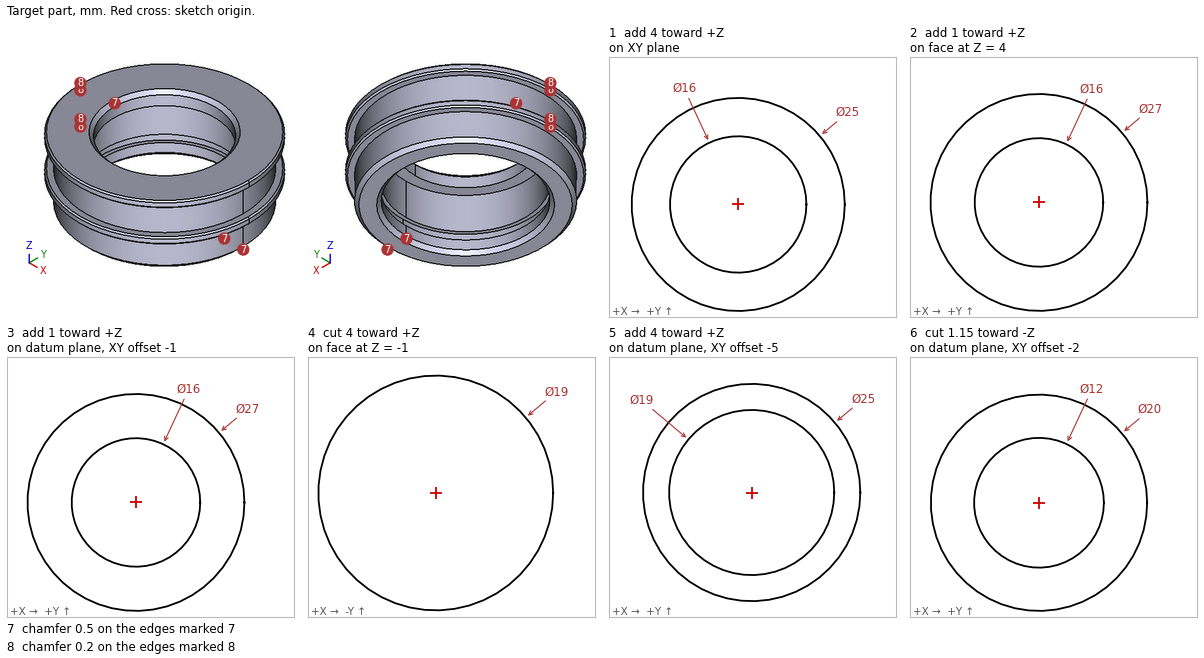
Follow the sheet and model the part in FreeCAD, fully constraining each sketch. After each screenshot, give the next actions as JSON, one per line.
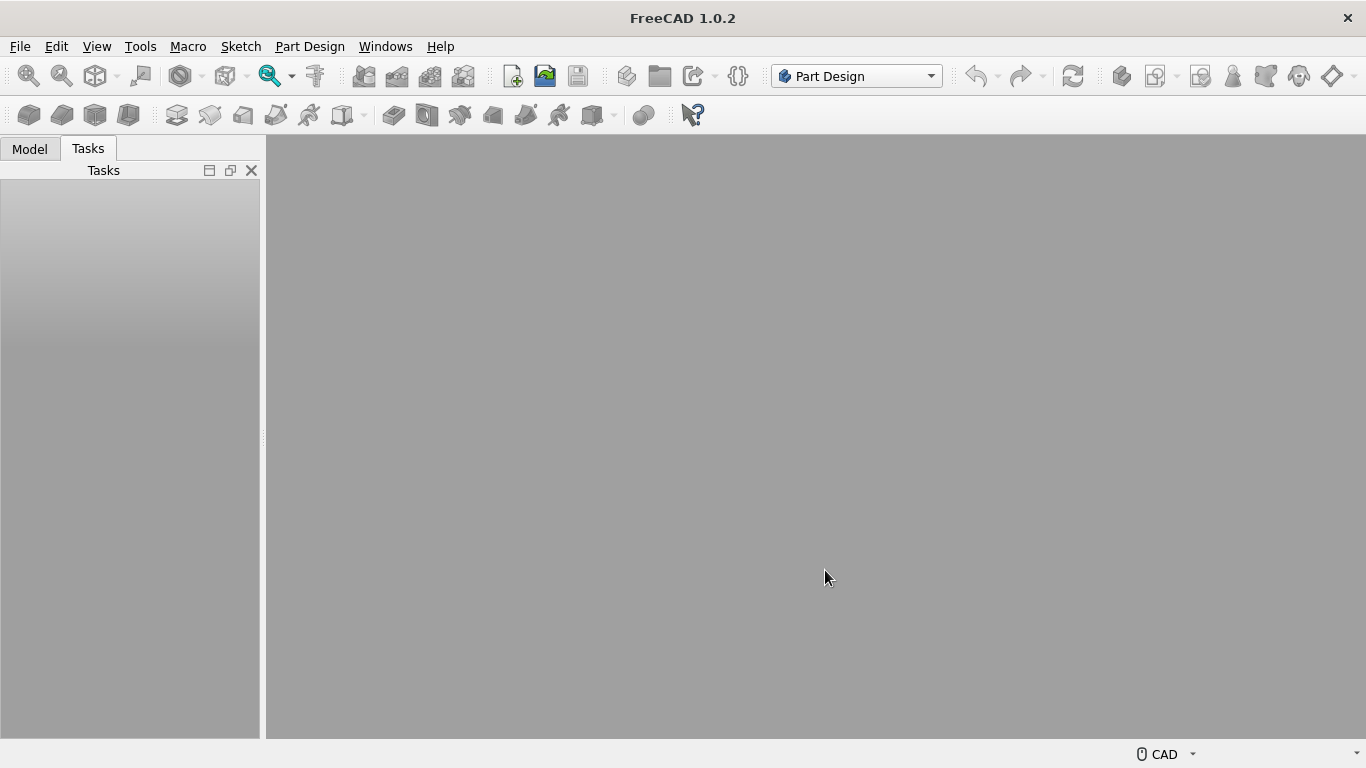
{"action": "left_click", "coordinate": [512, 76]}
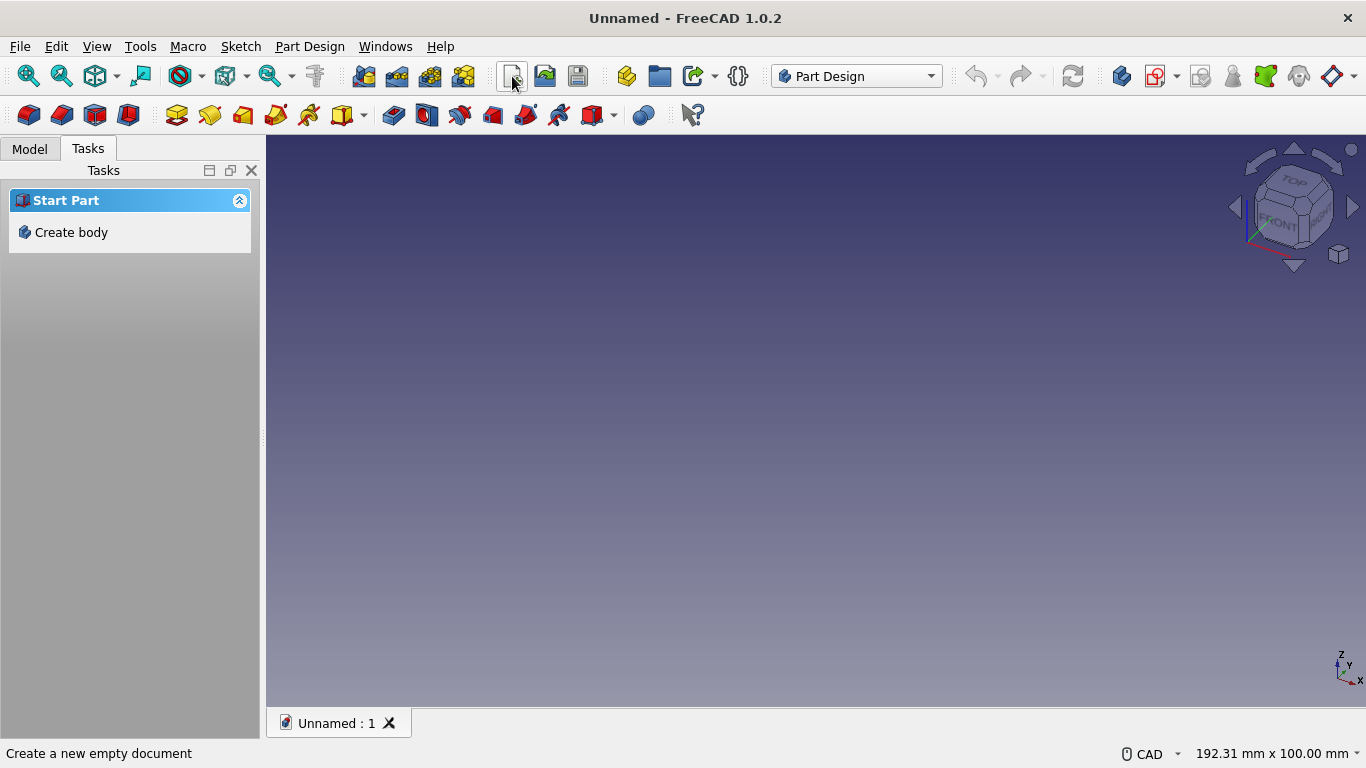
{"action": "left_click", "coordinate": [1154, 76]}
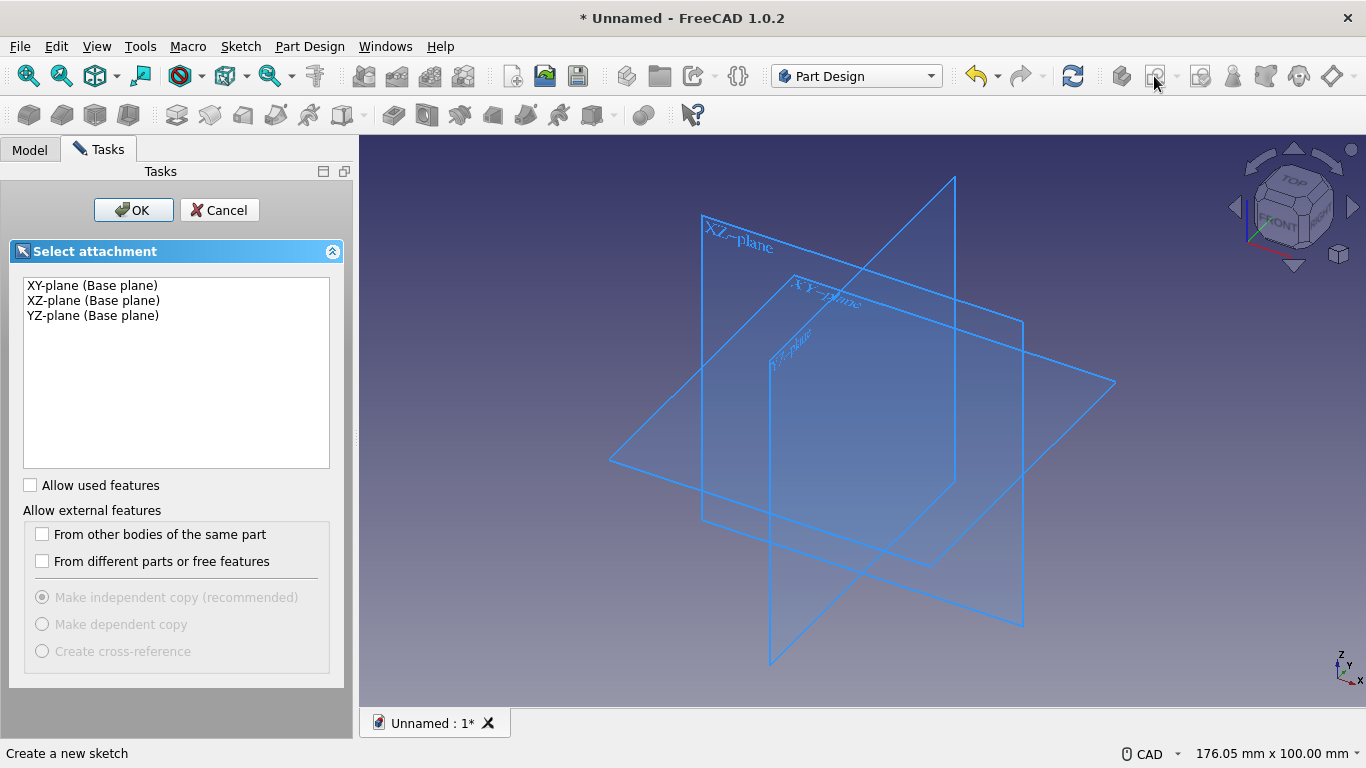
{"action": "left_click", "coordinate": [84, 286]}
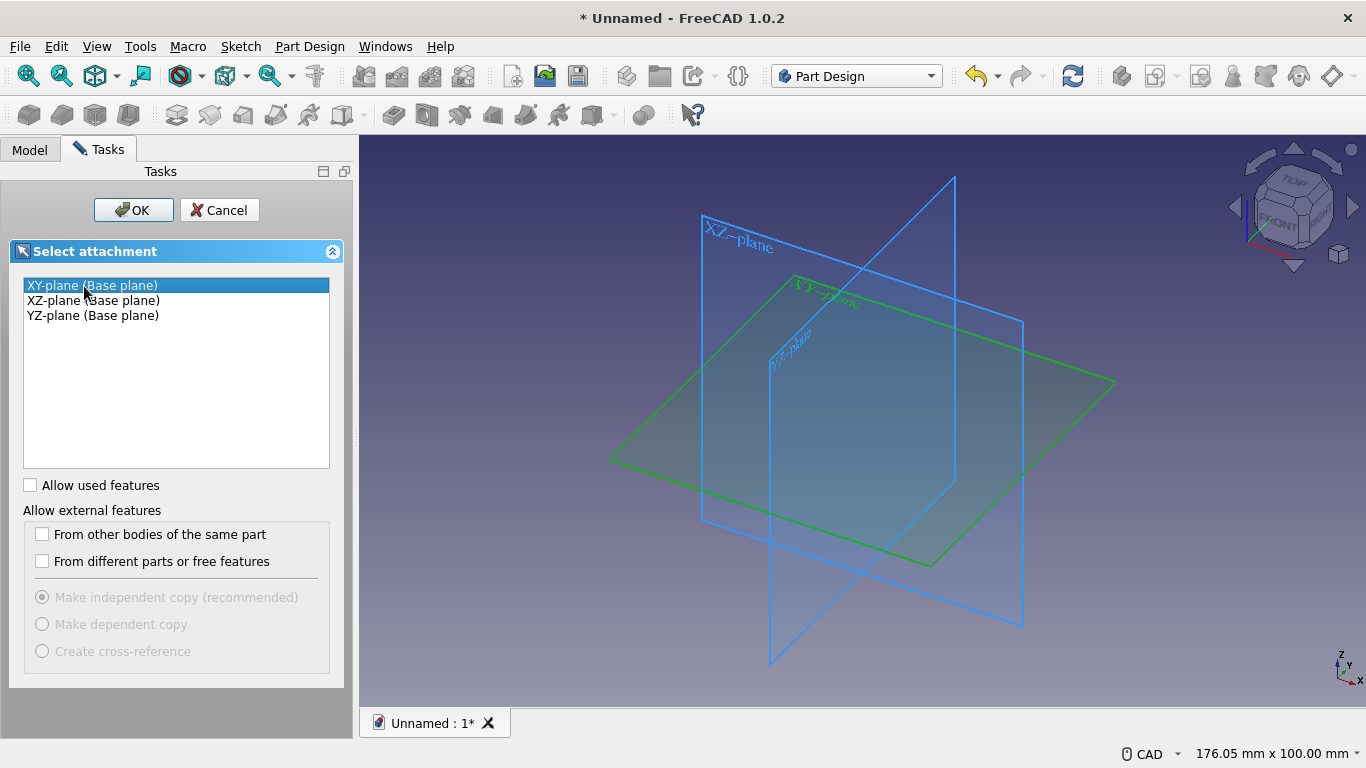
{"action": "left_click", "coordinate": [134, 210]}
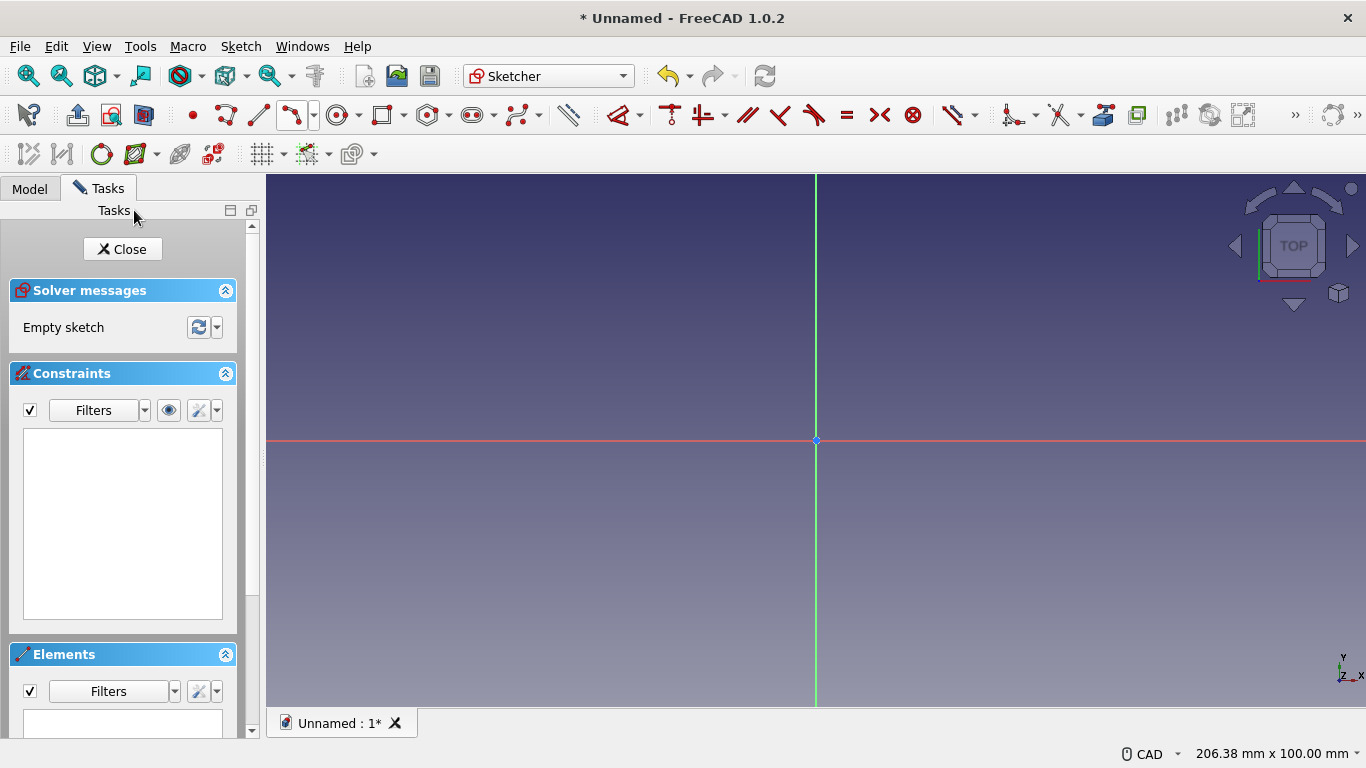
{"action": "scroll", "coordinate": [856, 440], "scroll_direction": "up", "scroll_amount": 5}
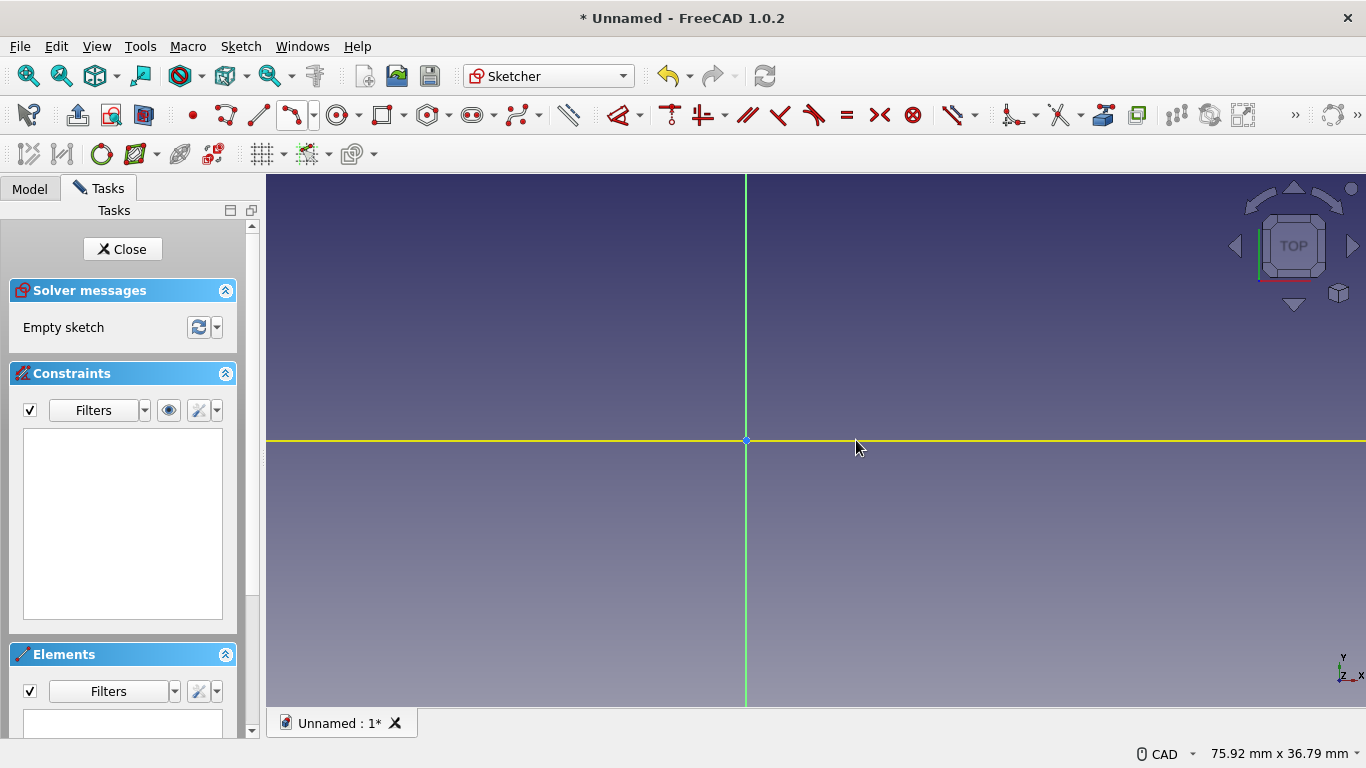
{"action": "left_click", "coordinate": [336, 116]}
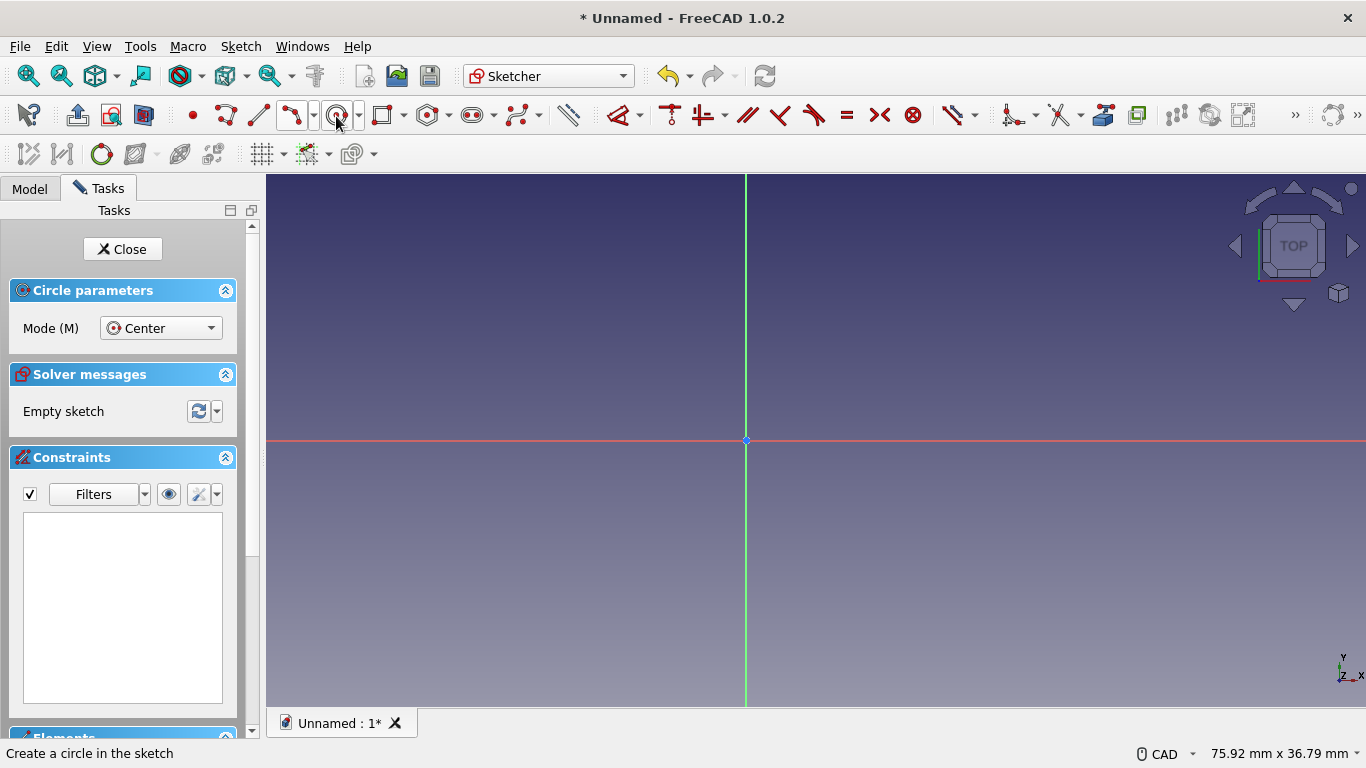
{"action": "left_click", "coordinate": [746, 440]}
{"action": "left_click", "coordinate": [874, 312]}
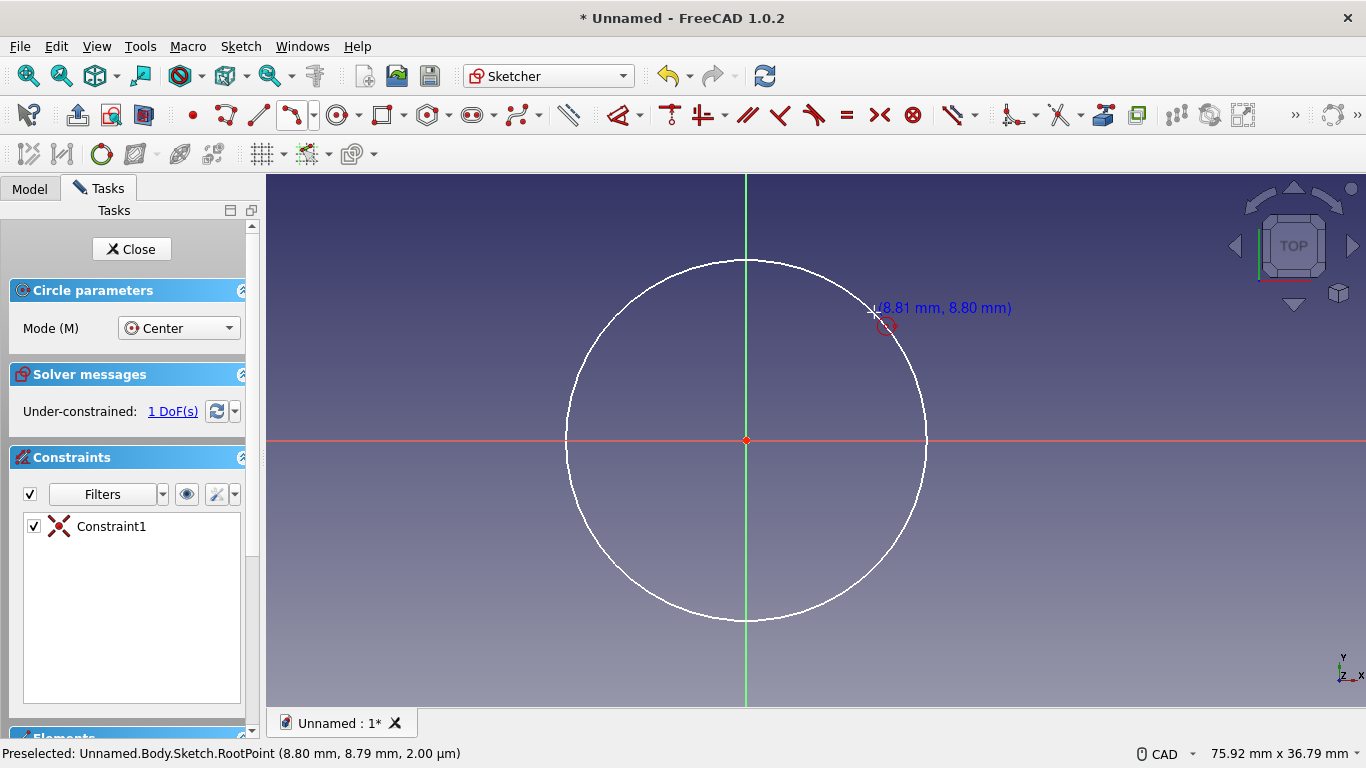
{"action": "left_click", "coordinate": [746, 440]}
{"action": "left_click", "coordinate": [828, 359]}
{"action": "key", "text": "Escape"}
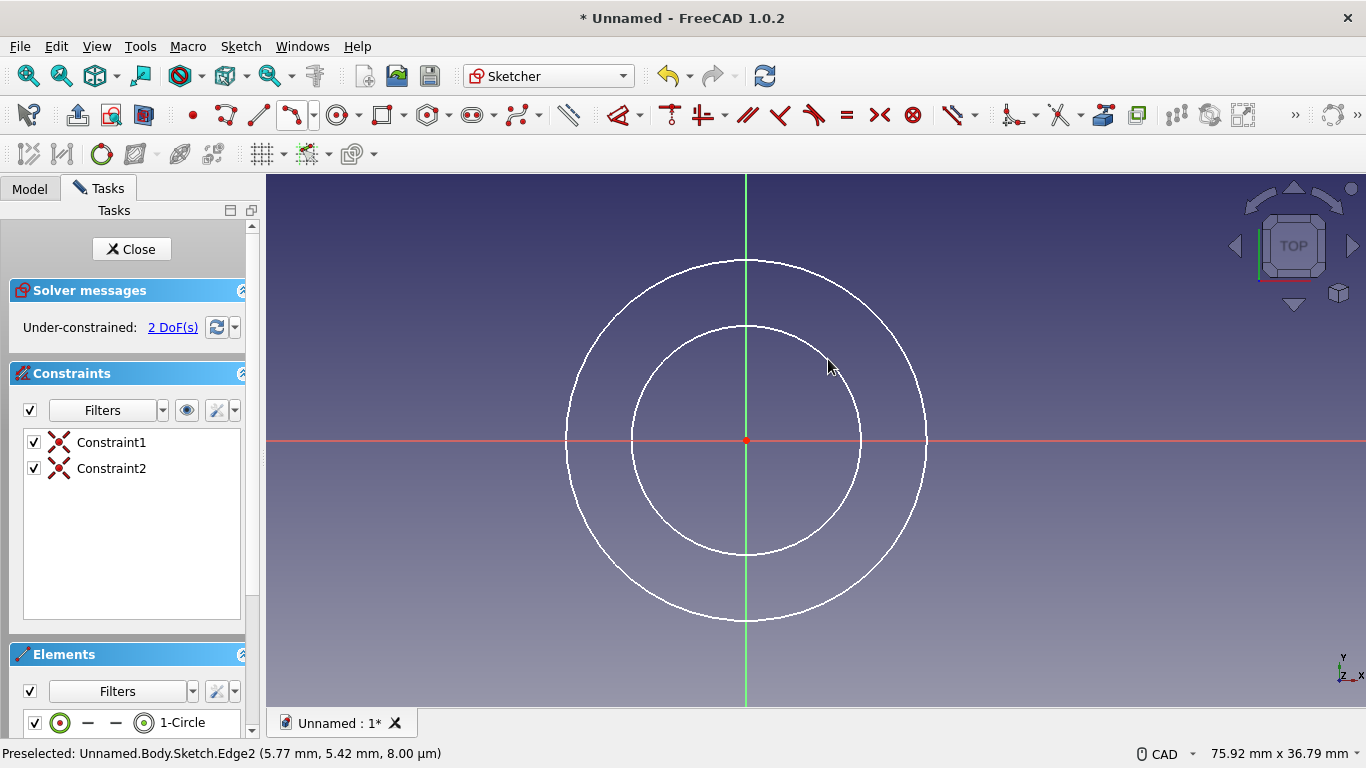
{"action": "left_click", "coordinate": [618, 116]}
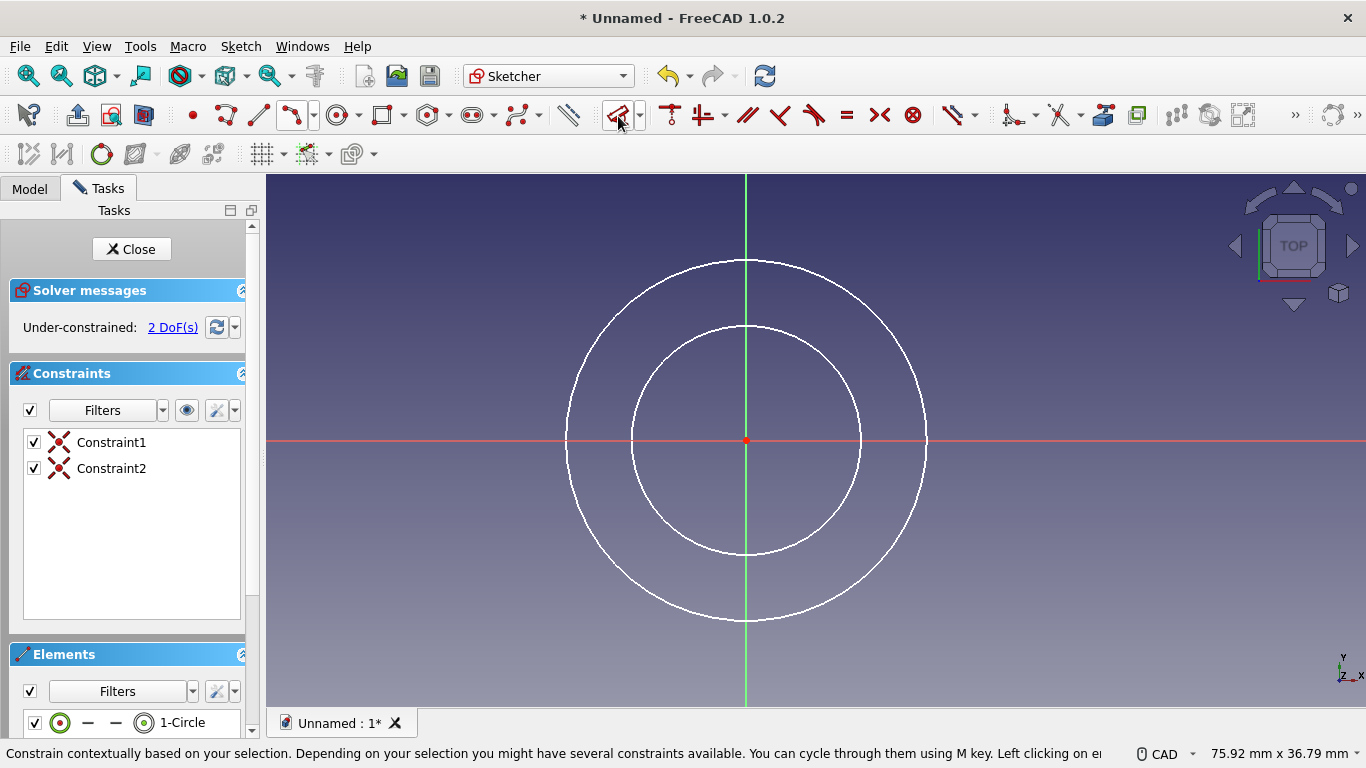
{"action": "left_click", "coordinate": [874, 313]}
{"action": "left_click", "coordinate": [897, 290]}